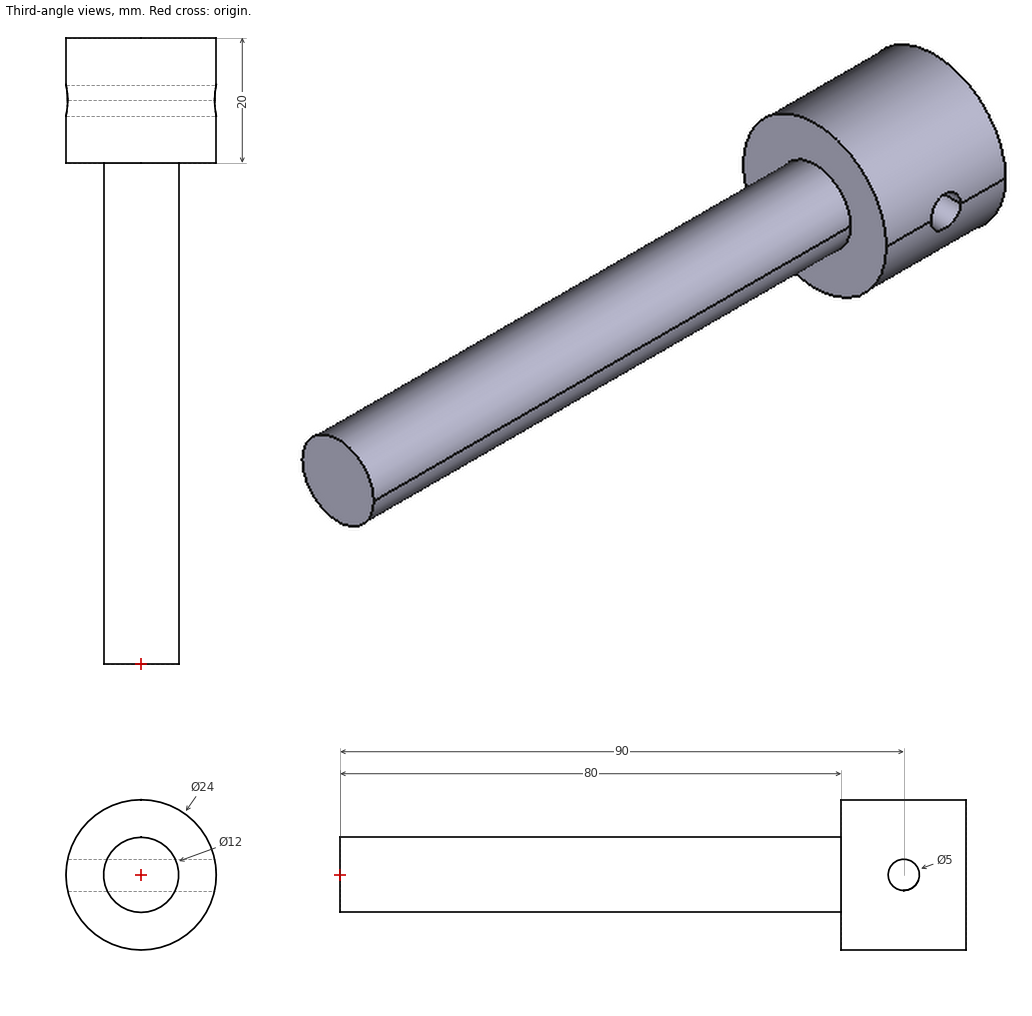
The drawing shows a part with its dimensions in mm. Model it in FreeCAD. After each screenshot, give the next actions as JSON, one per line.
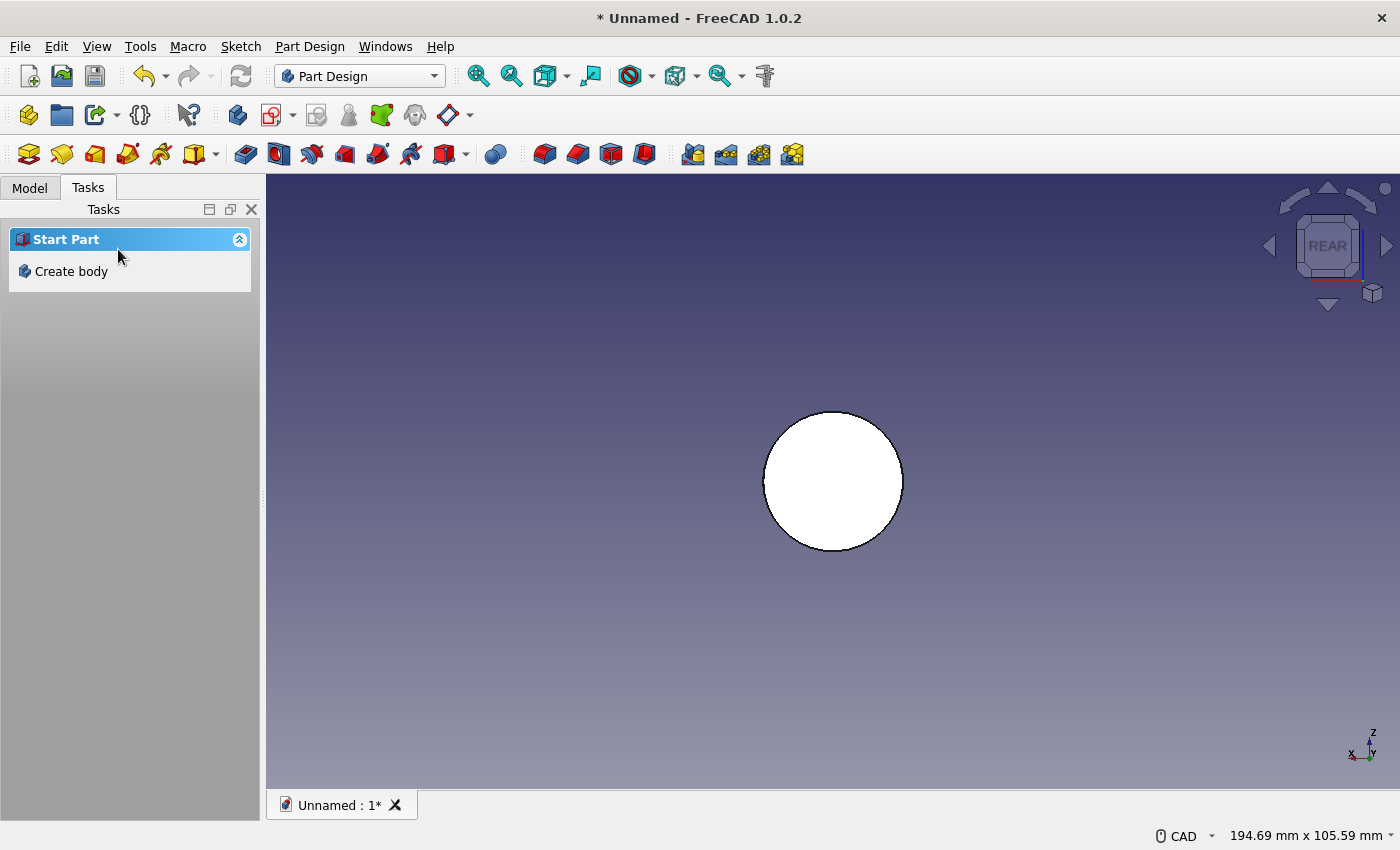
{"action": "key", "text": "0"}